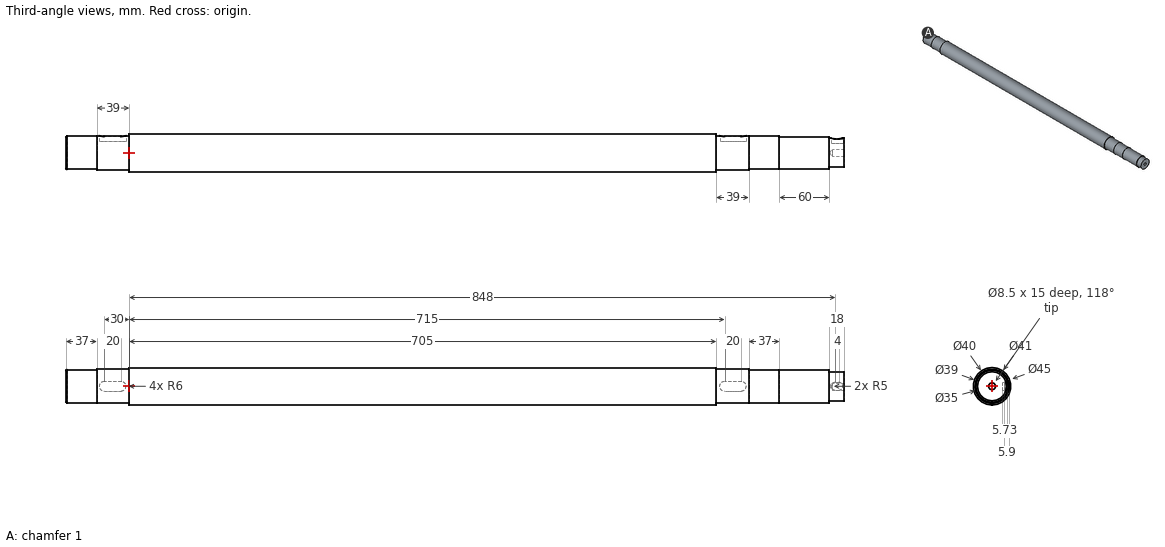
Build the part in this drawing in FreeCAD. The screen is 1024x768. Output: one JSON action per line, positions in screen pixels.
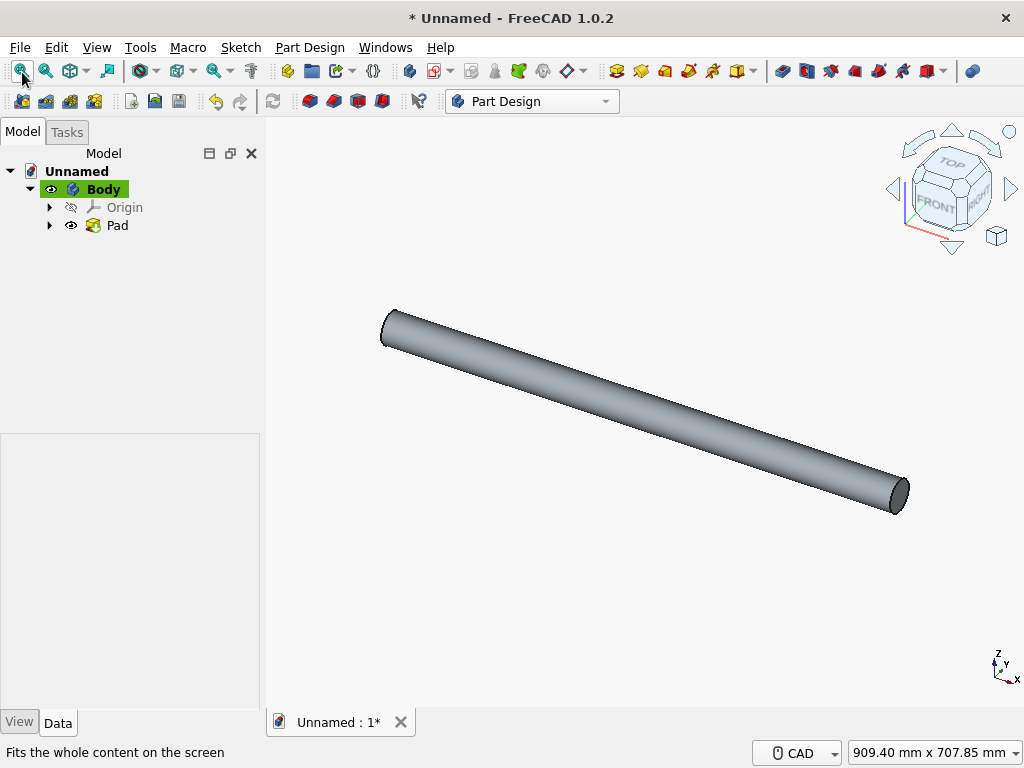
{"action": "left_click", "coordinate": [902, 493]}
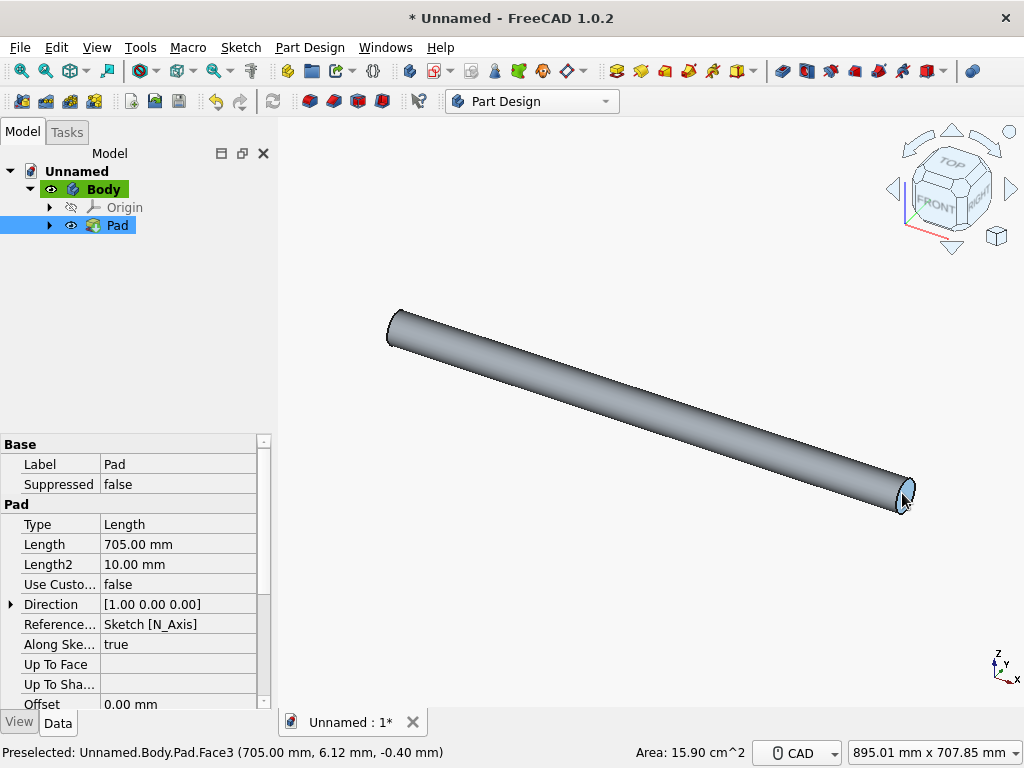
{"action": "left_click", "coordinate": [434, 72]}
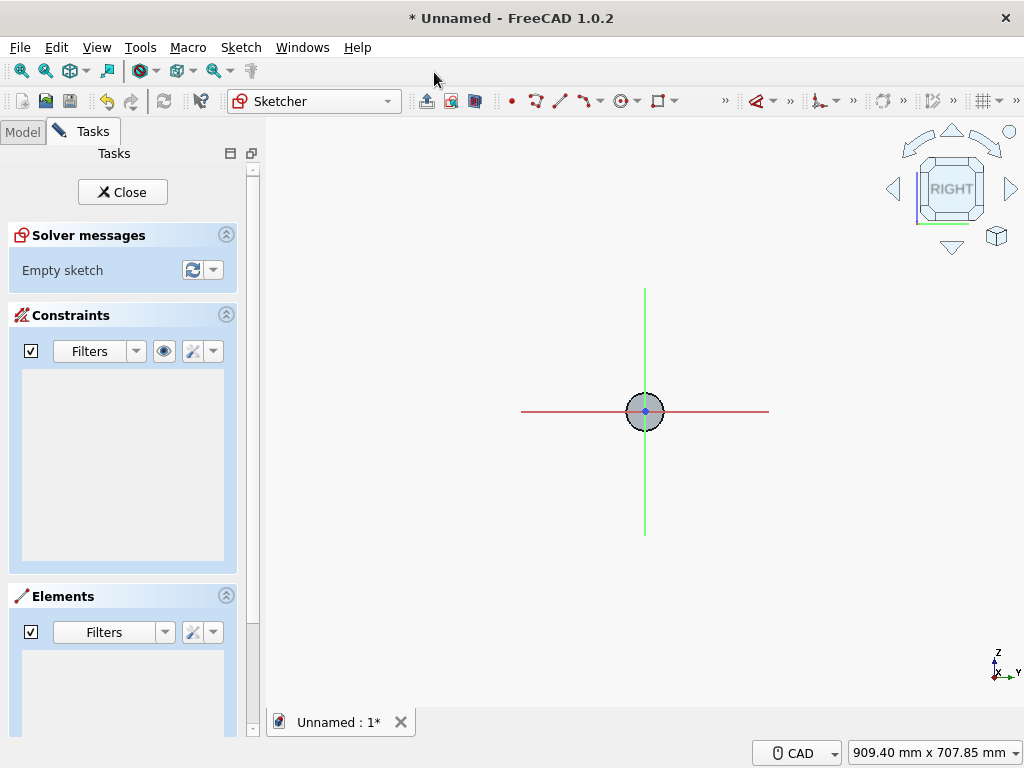
{"action": "scroll", "coordinate": [652, 412], "scroll_direction": "up", "scroll_amount": 12}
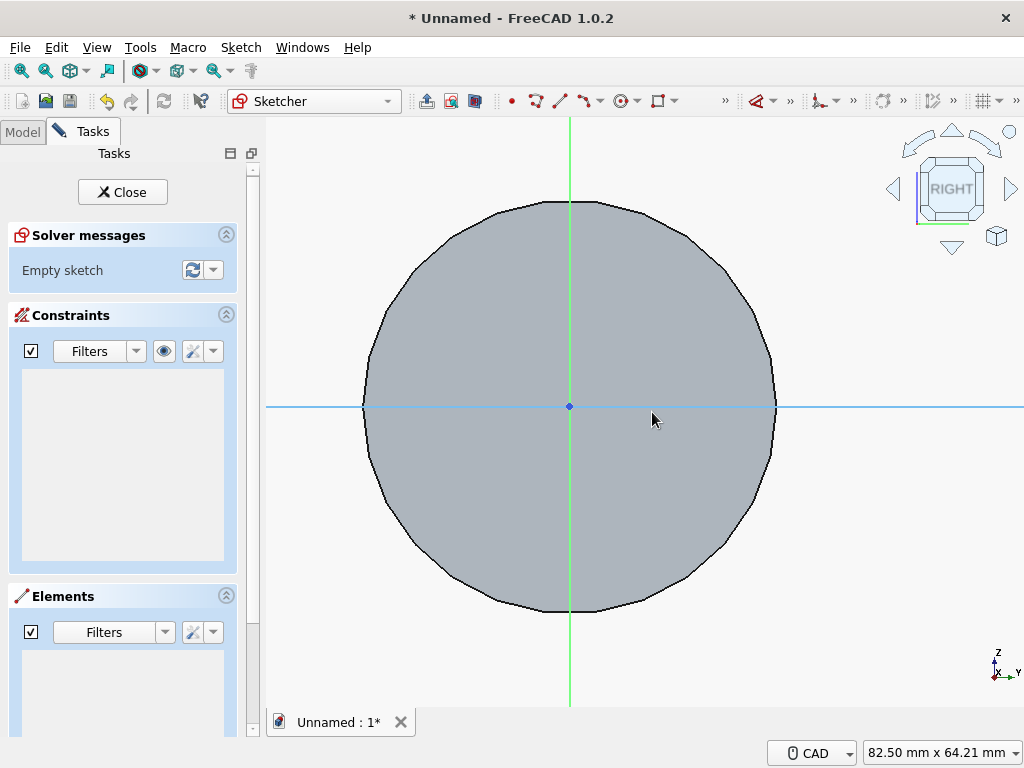
{"action": "left_click", "coordinate": [622, 102]}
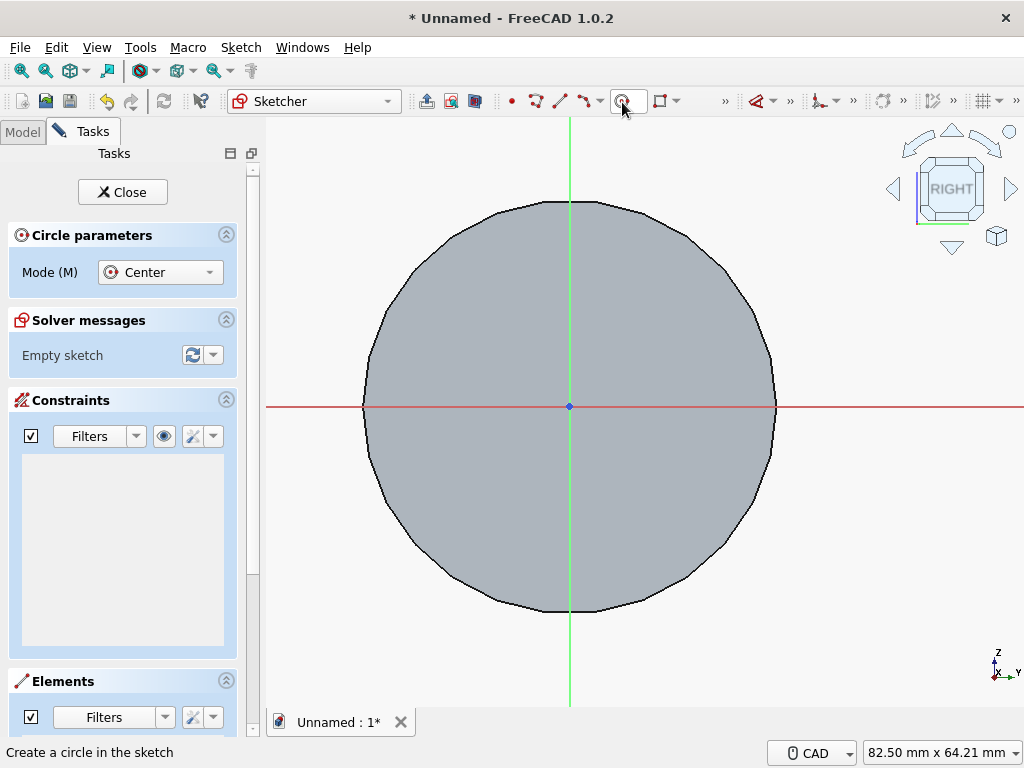
{"action": "left_click", "coordinate": [570, 407]}
{"action": "mouse_move", "coordinate": [703, 274]}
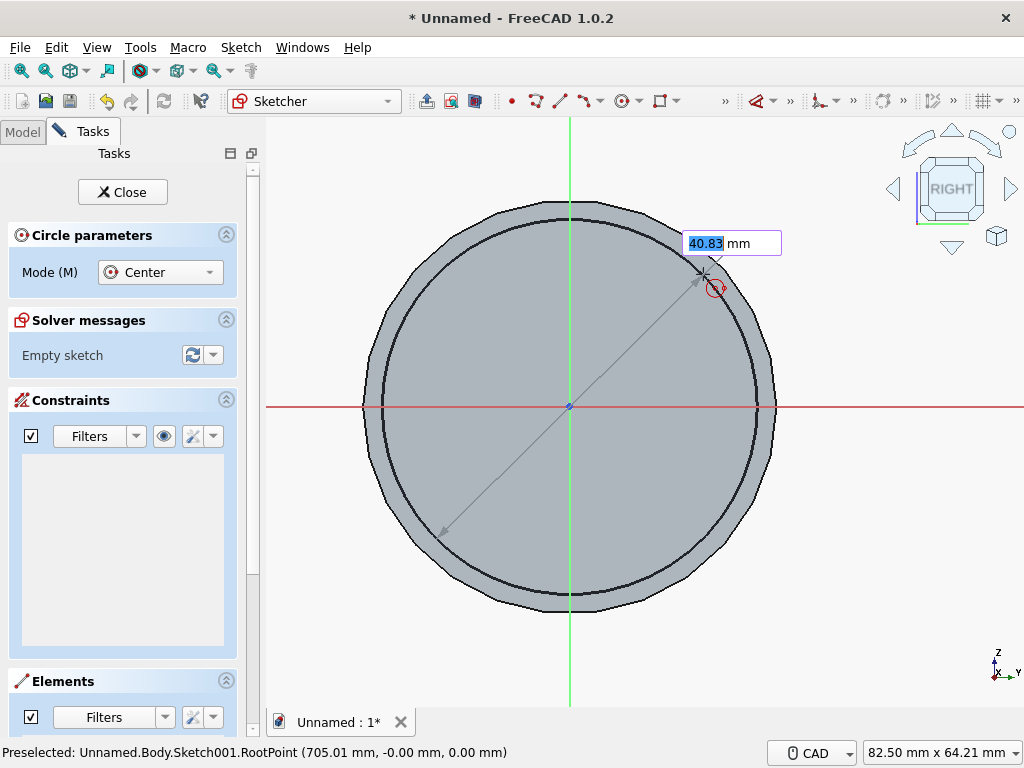
{"action": "type", "text": "41"}
{"action": "key", "text": "Return"}
{"action": "key", "text": "Escape"}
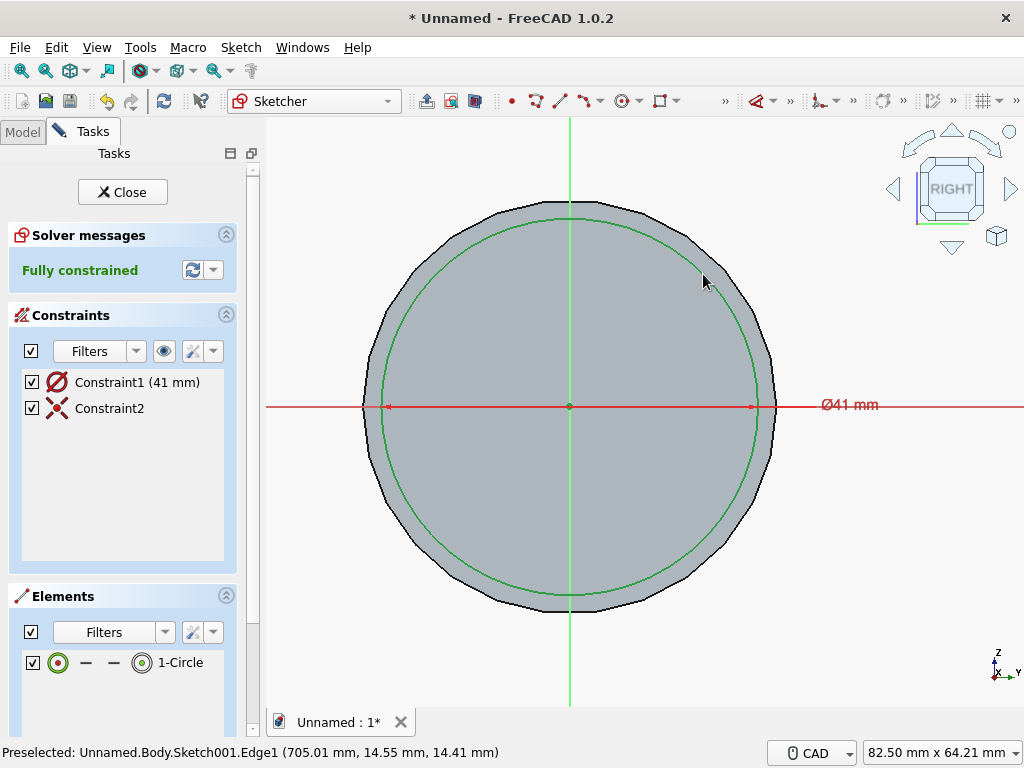
{"action": "left_click", "coordinate": [123, 192]}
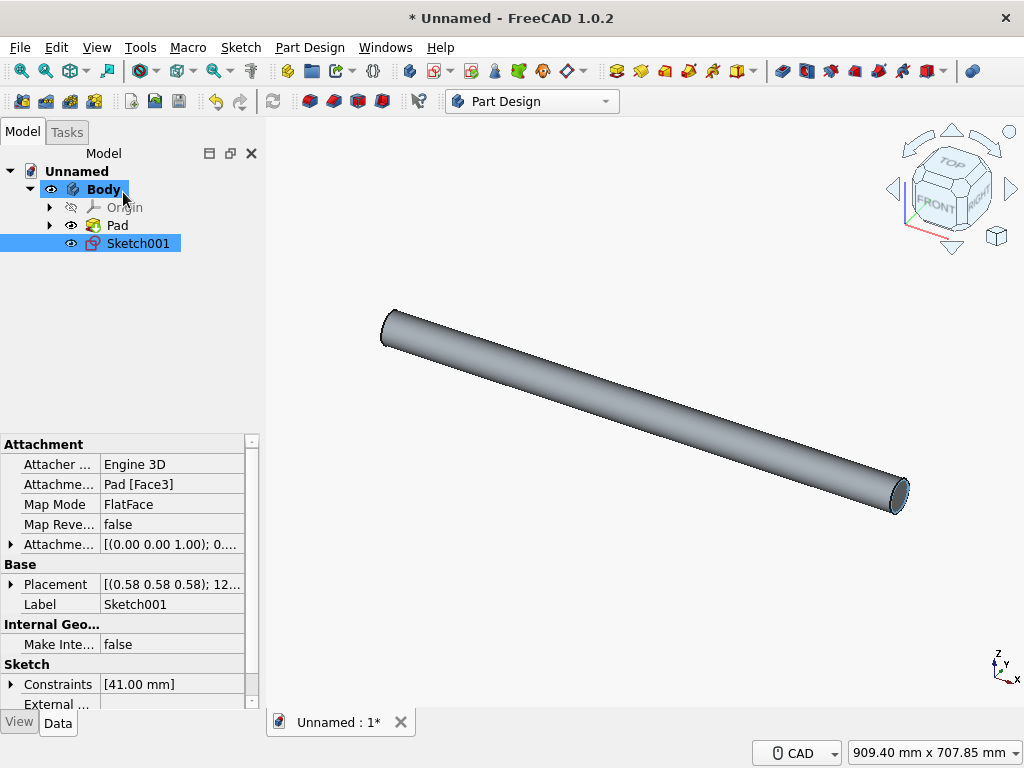
{"action": "left_click", "coordinate": [618, 72]}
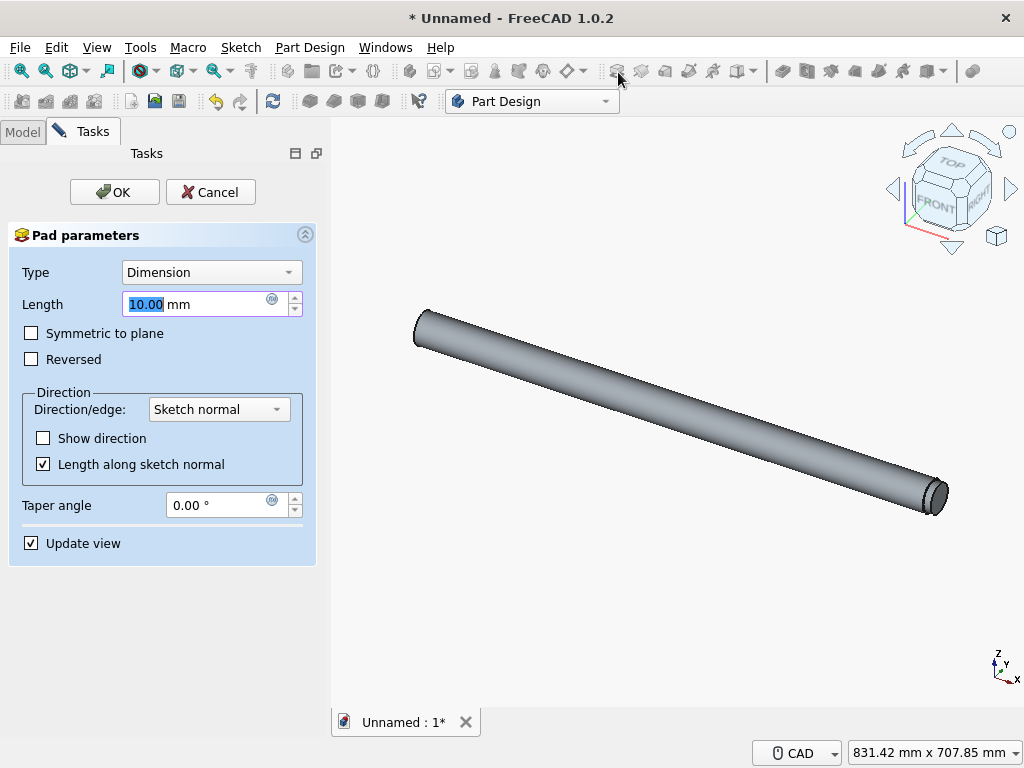
{"action": "type", "text": "39"}
{"action": "key", "text": "Tab"}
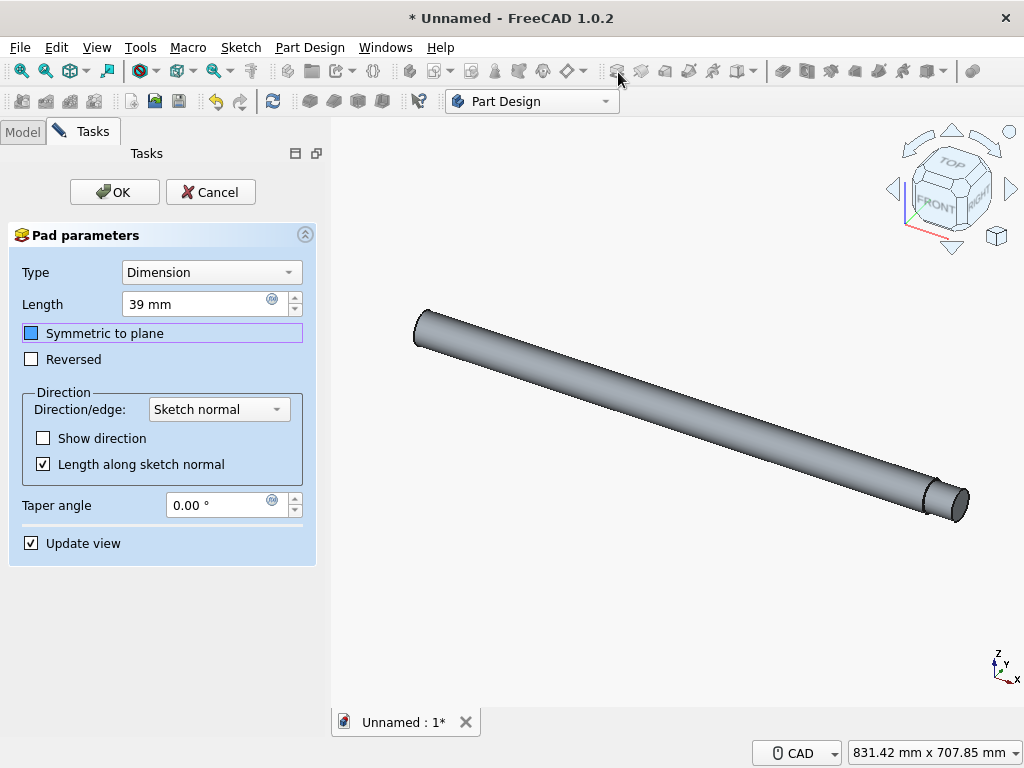
{"action": "left_click", "coordinate": [115, 192]}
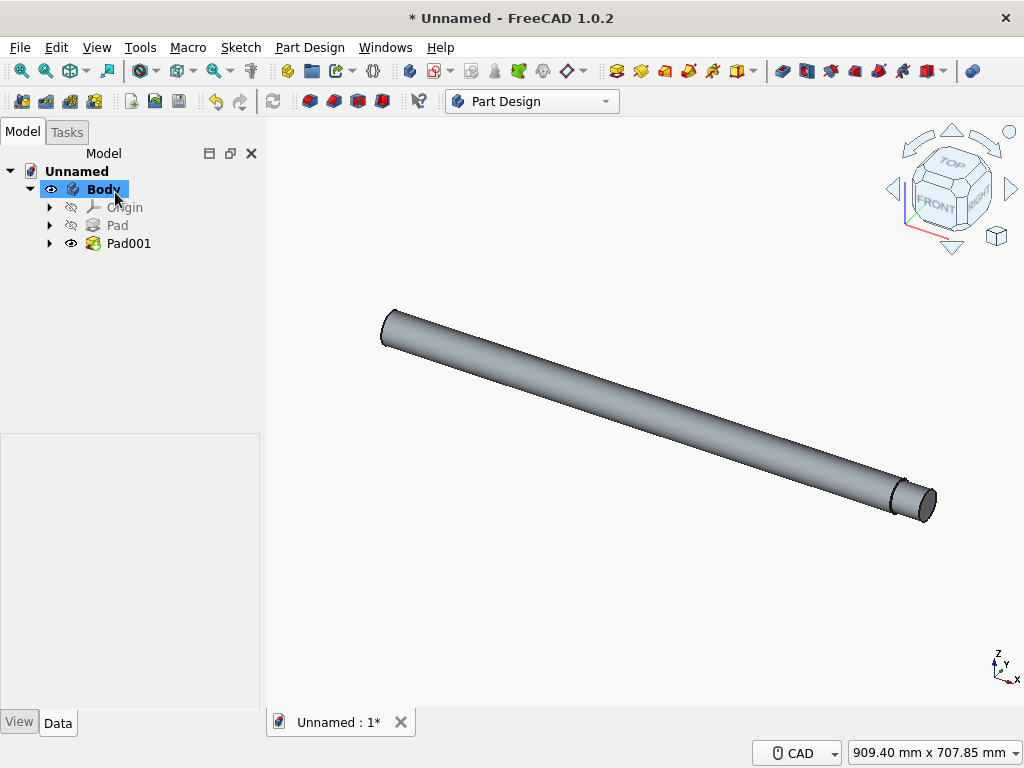
{"action": "left_click", "coordinate": [930, 506]}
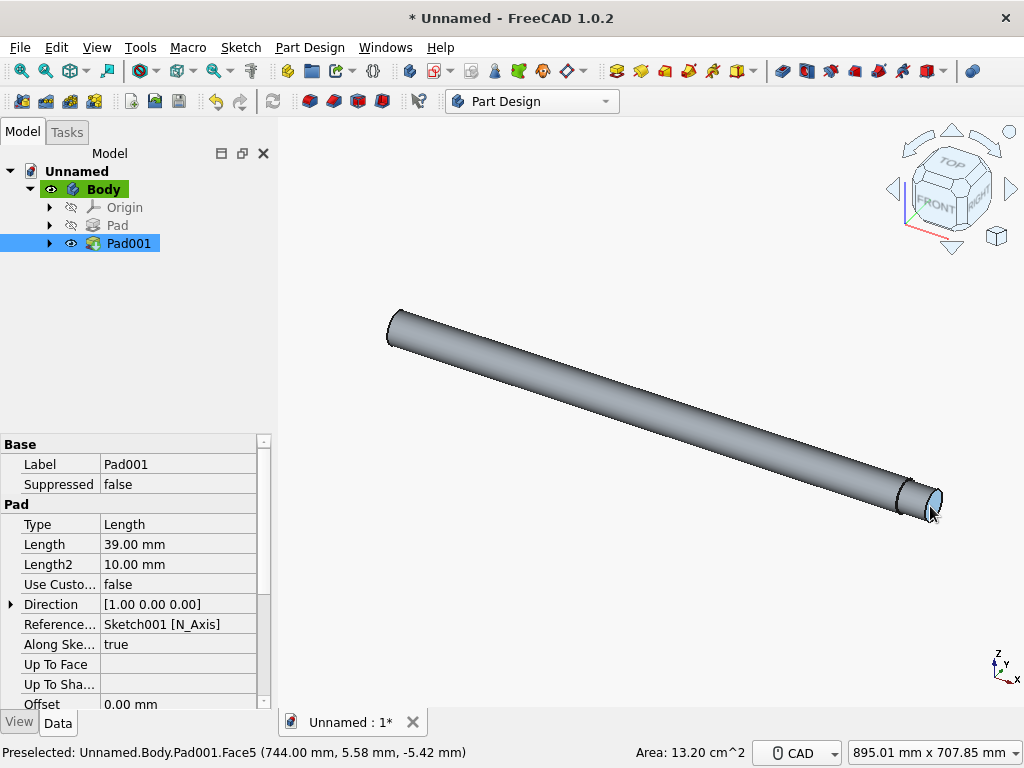
{"action": "left_click", "coordinate": [434, 72]}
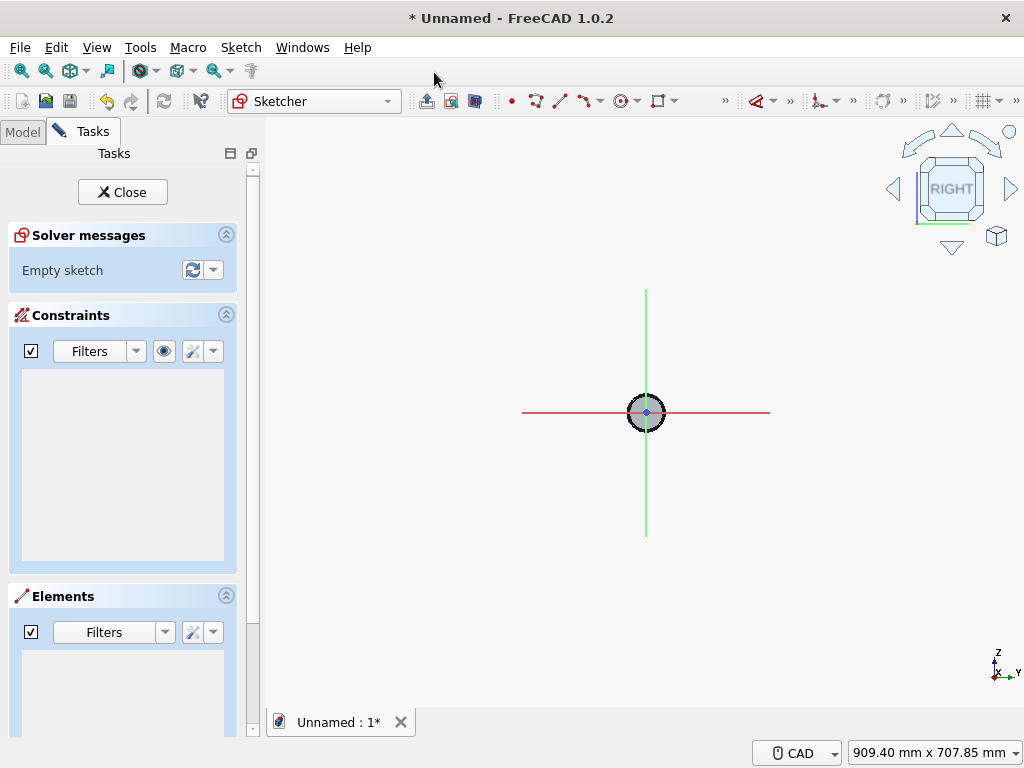
{"action": "scroll", "coordinate": [653, 413], "scroll_direction": "up", "scroll_amount": 12}